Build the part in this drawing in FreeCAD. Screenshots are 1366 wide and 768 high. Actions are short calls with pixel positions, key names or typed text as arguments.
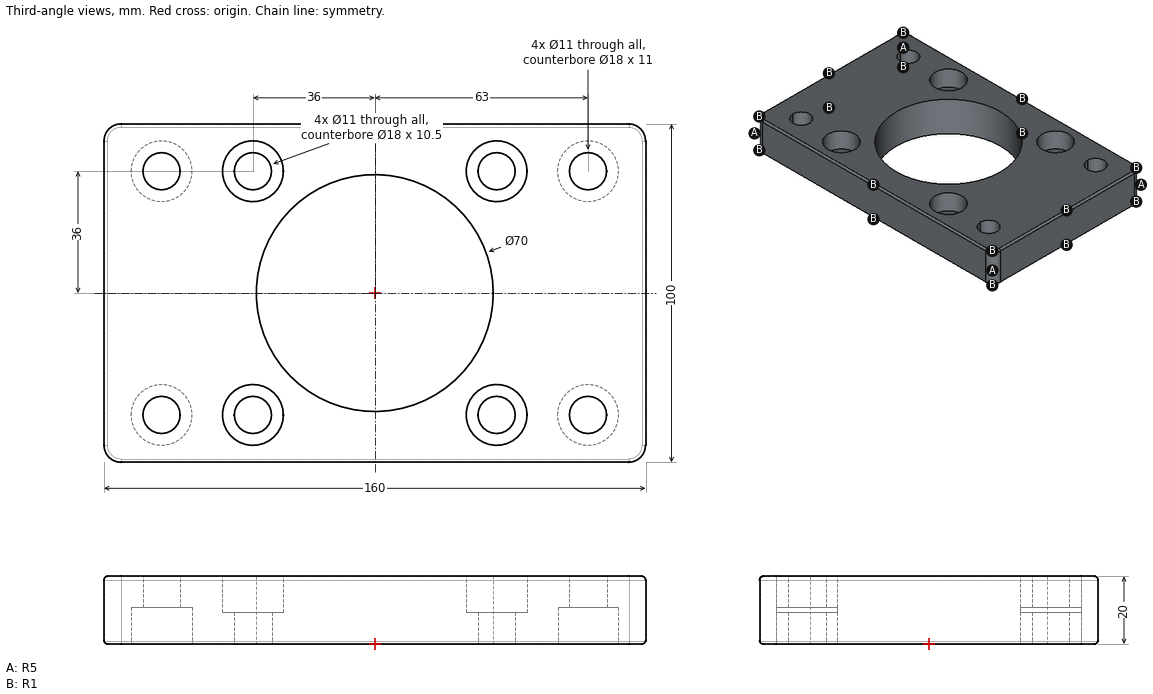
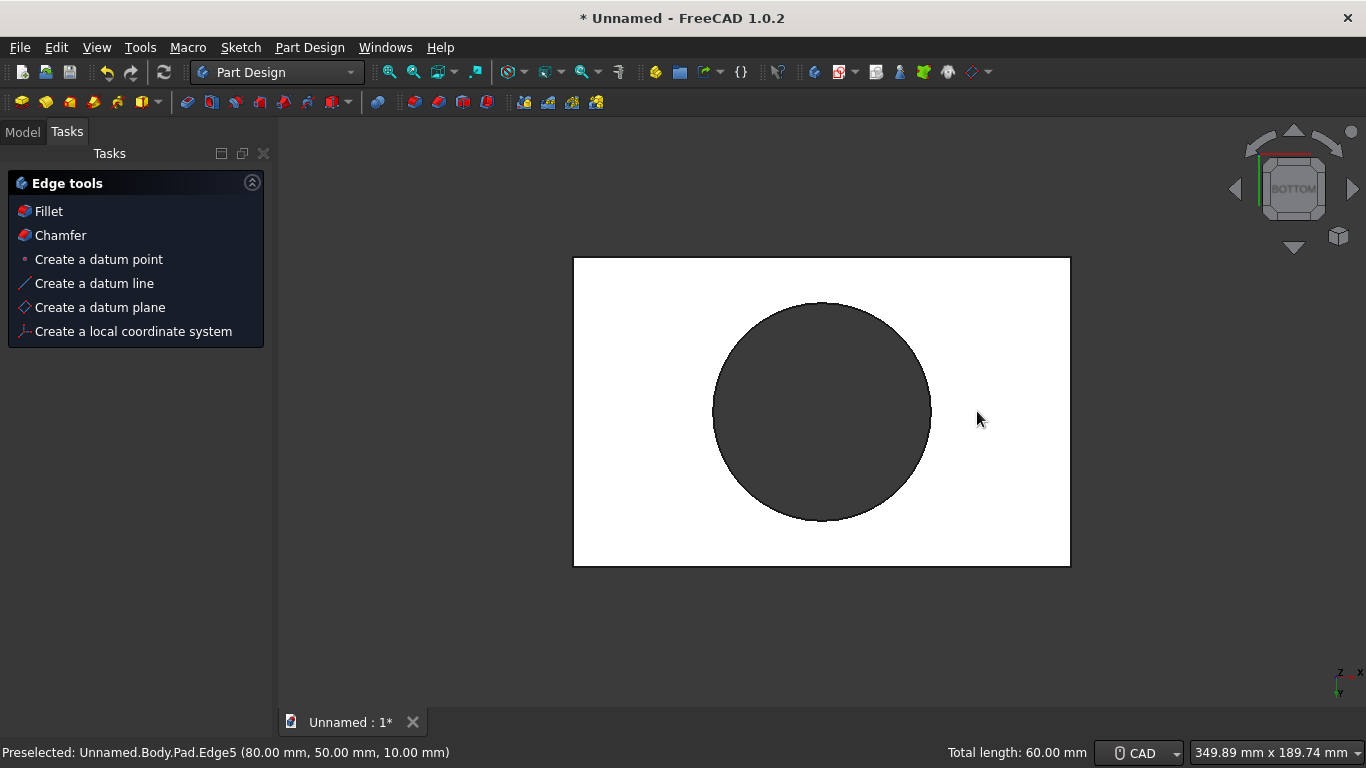
key(4)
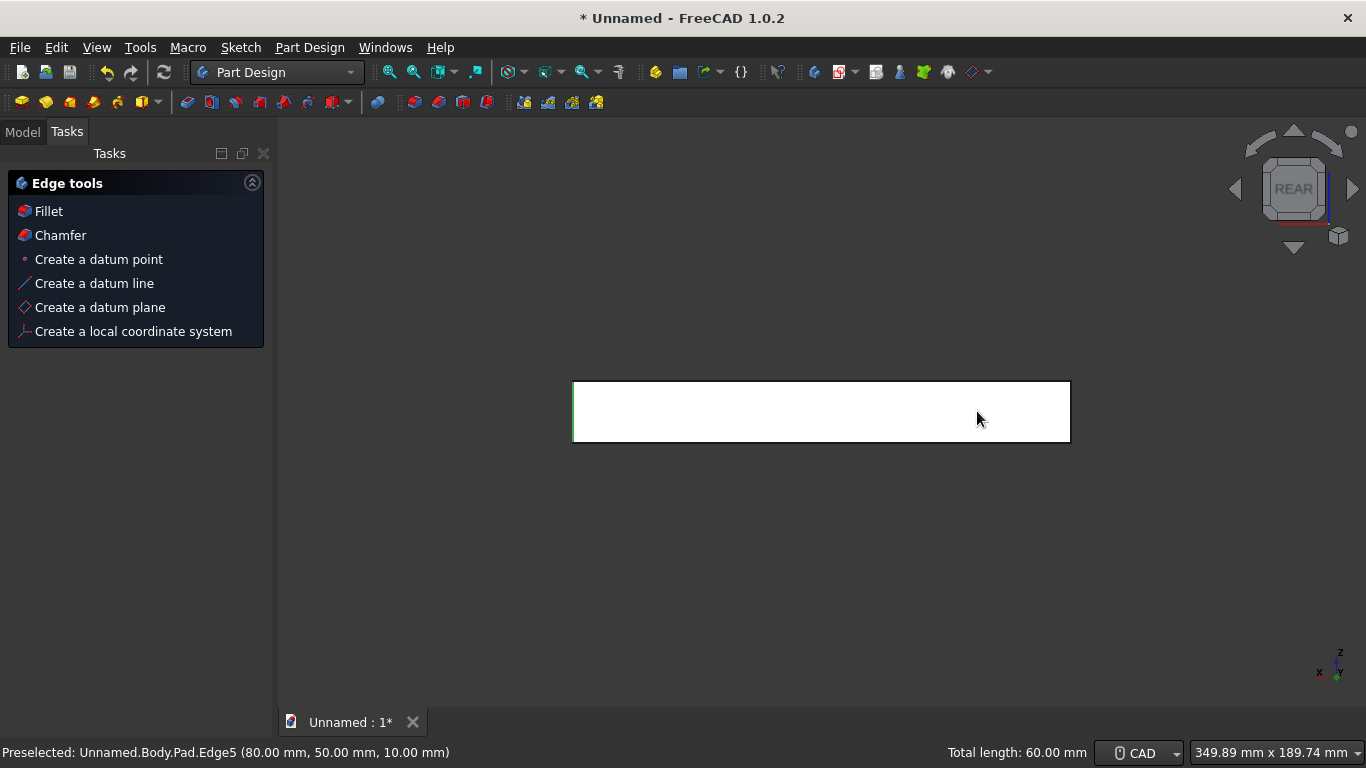
click(1071, 411, ctrl)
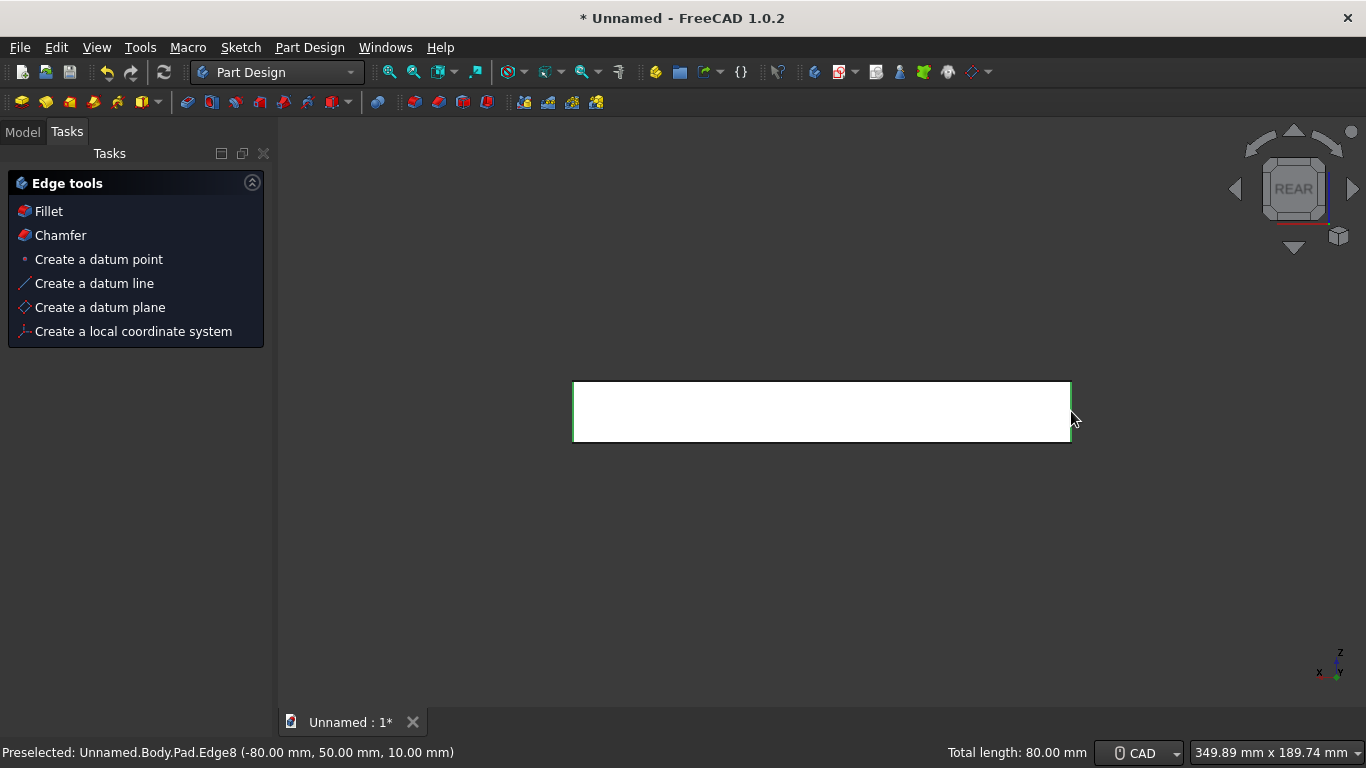
click(416, 102)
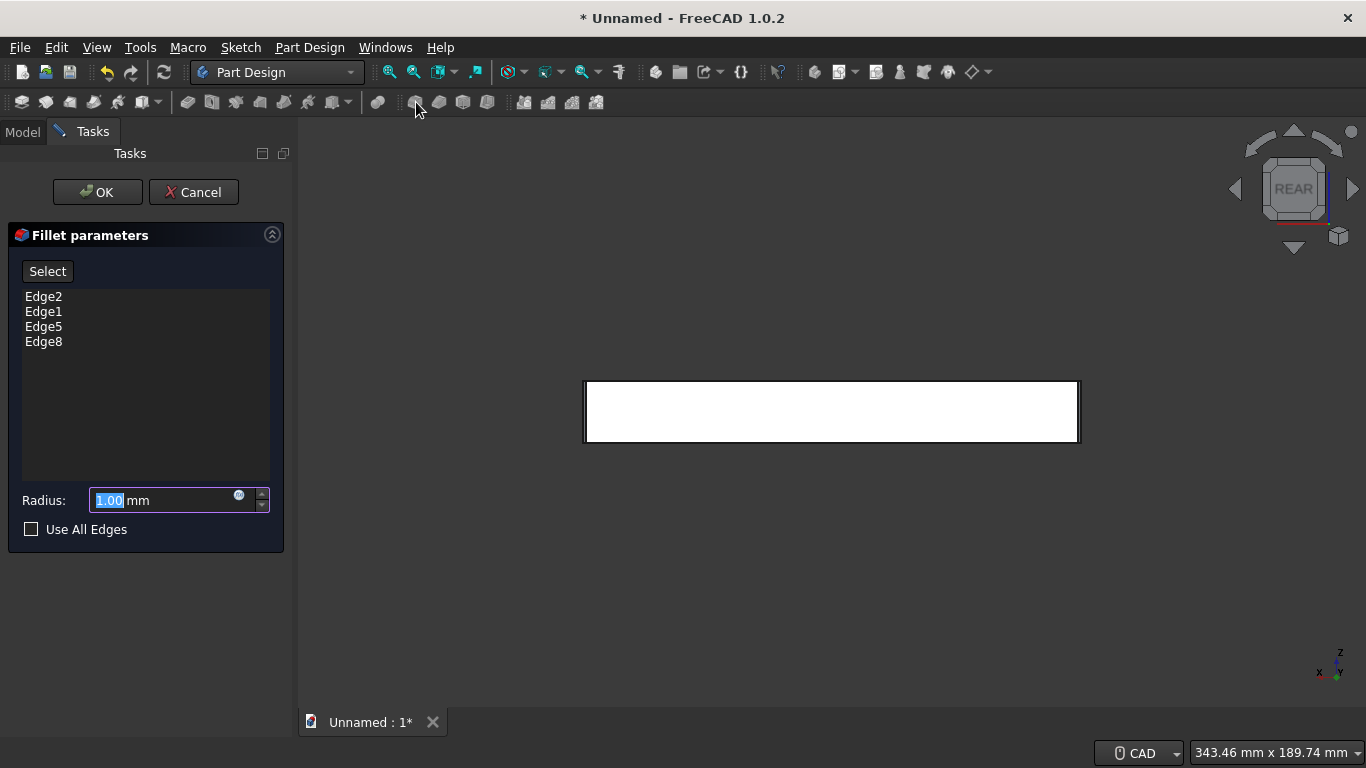
text(5)
key(Tab)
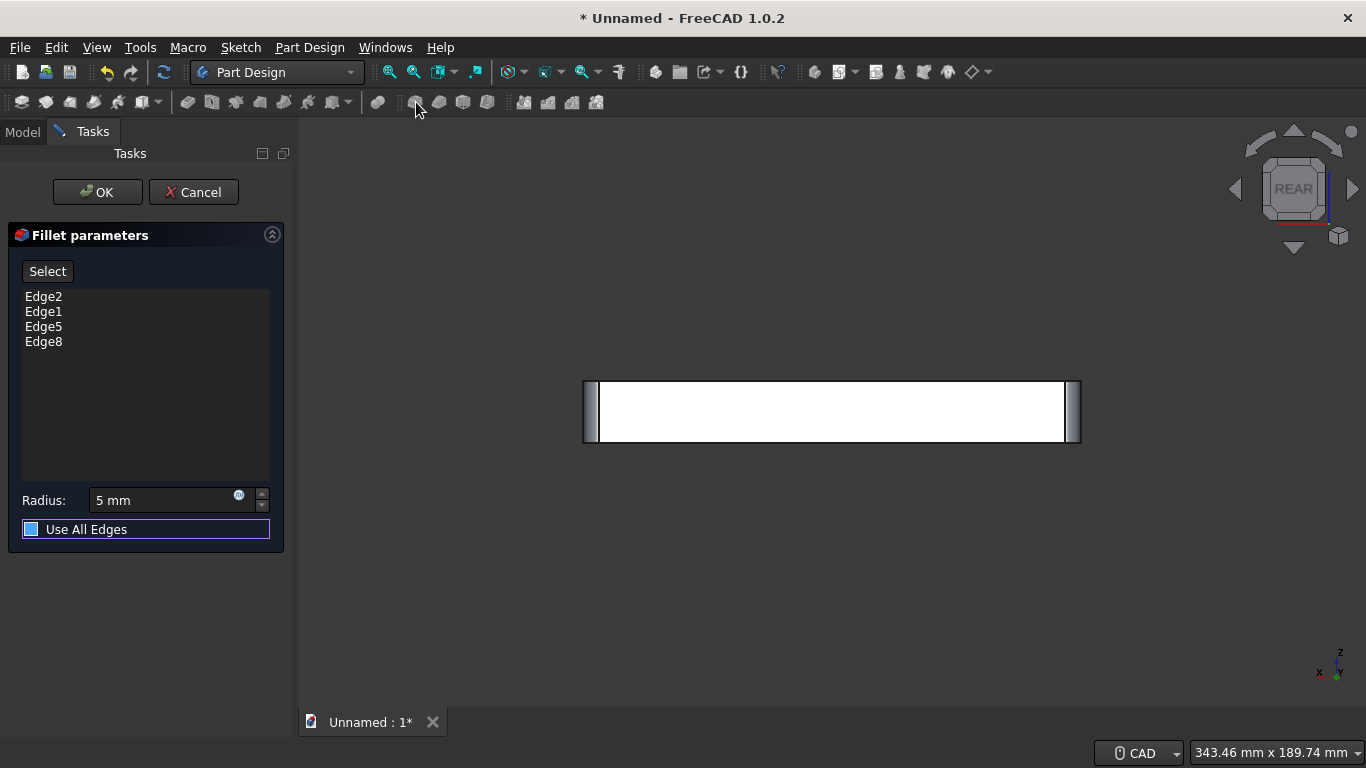
click(98, 192)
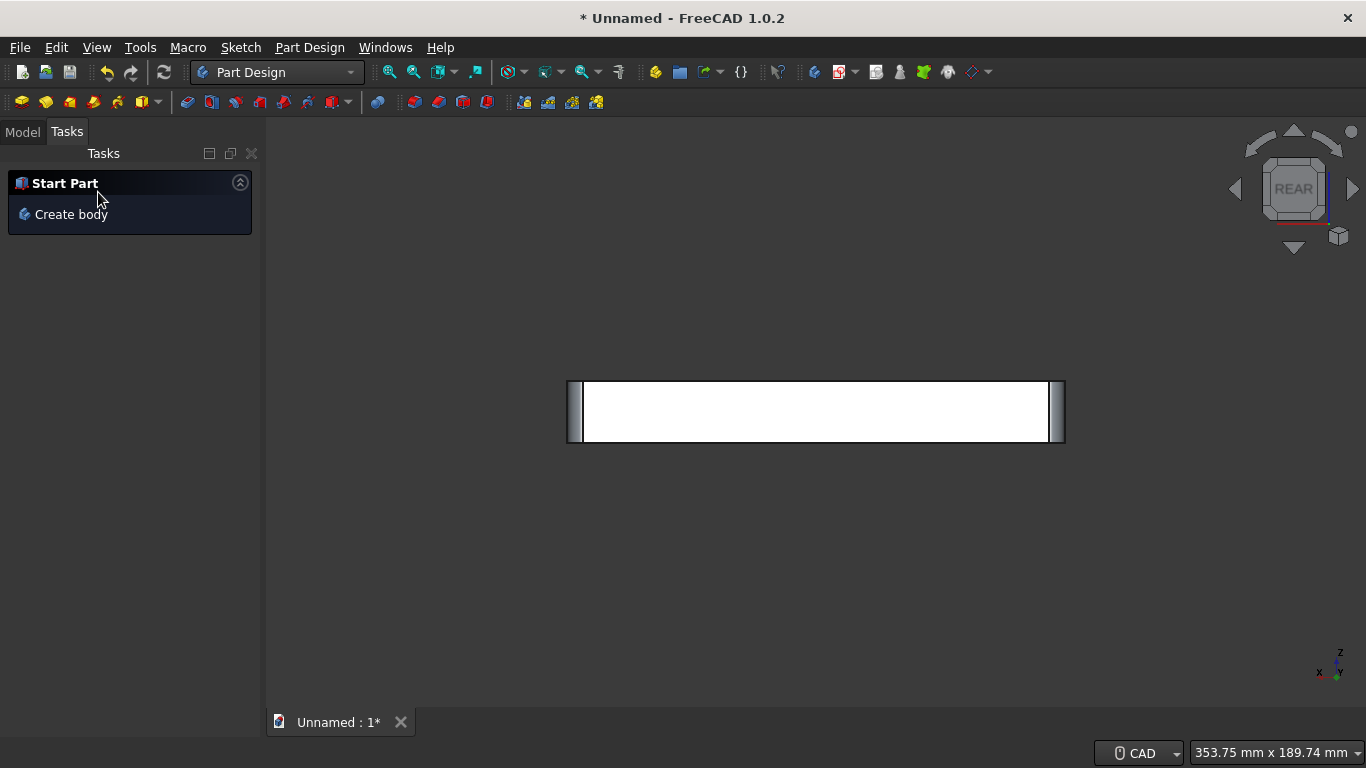
key(0)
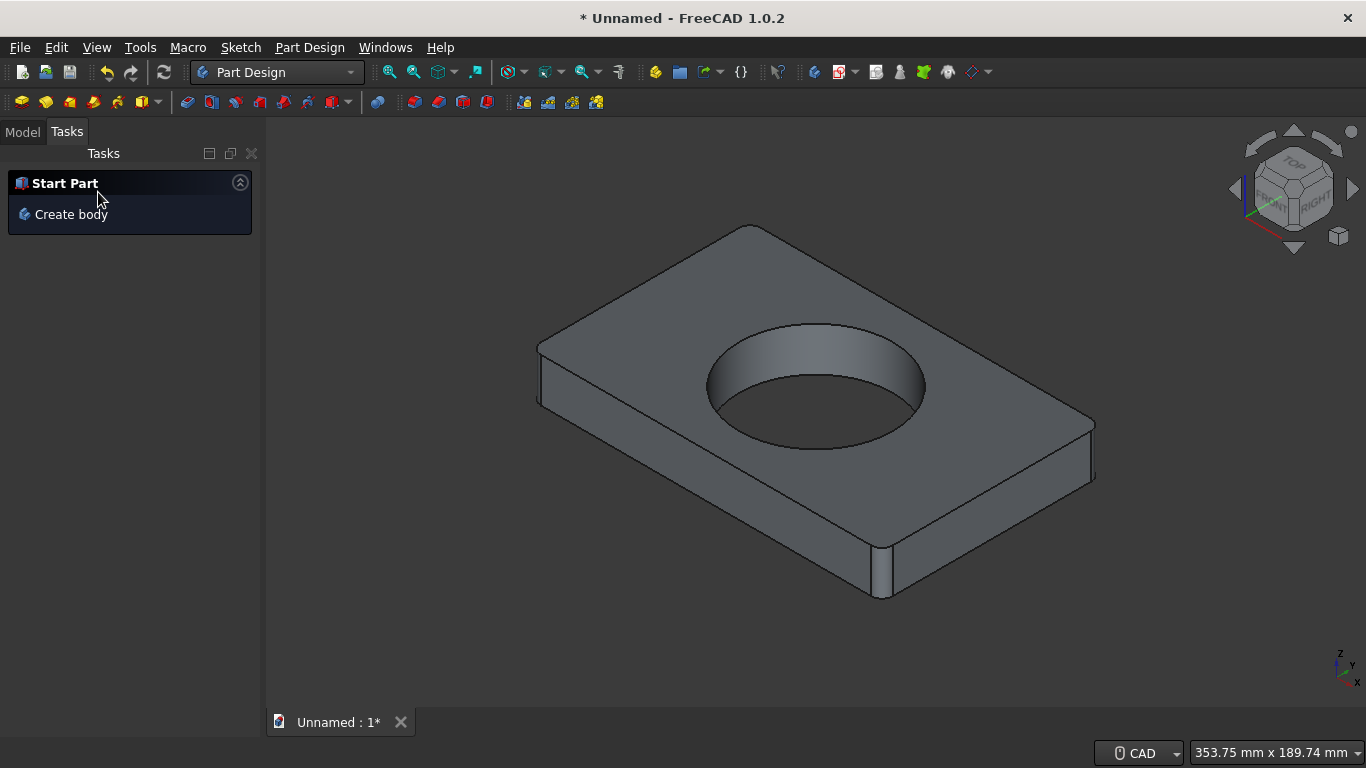
click(653, 364)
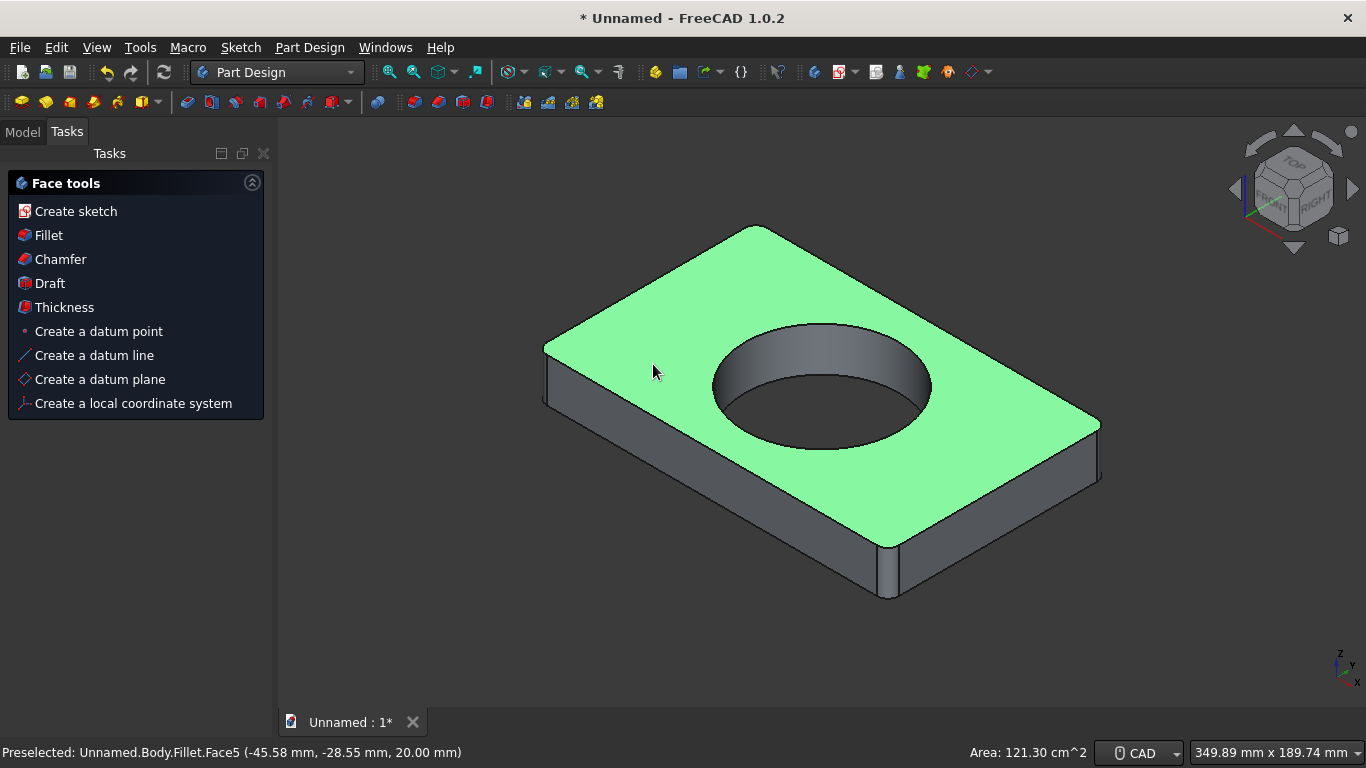
click(840, 72)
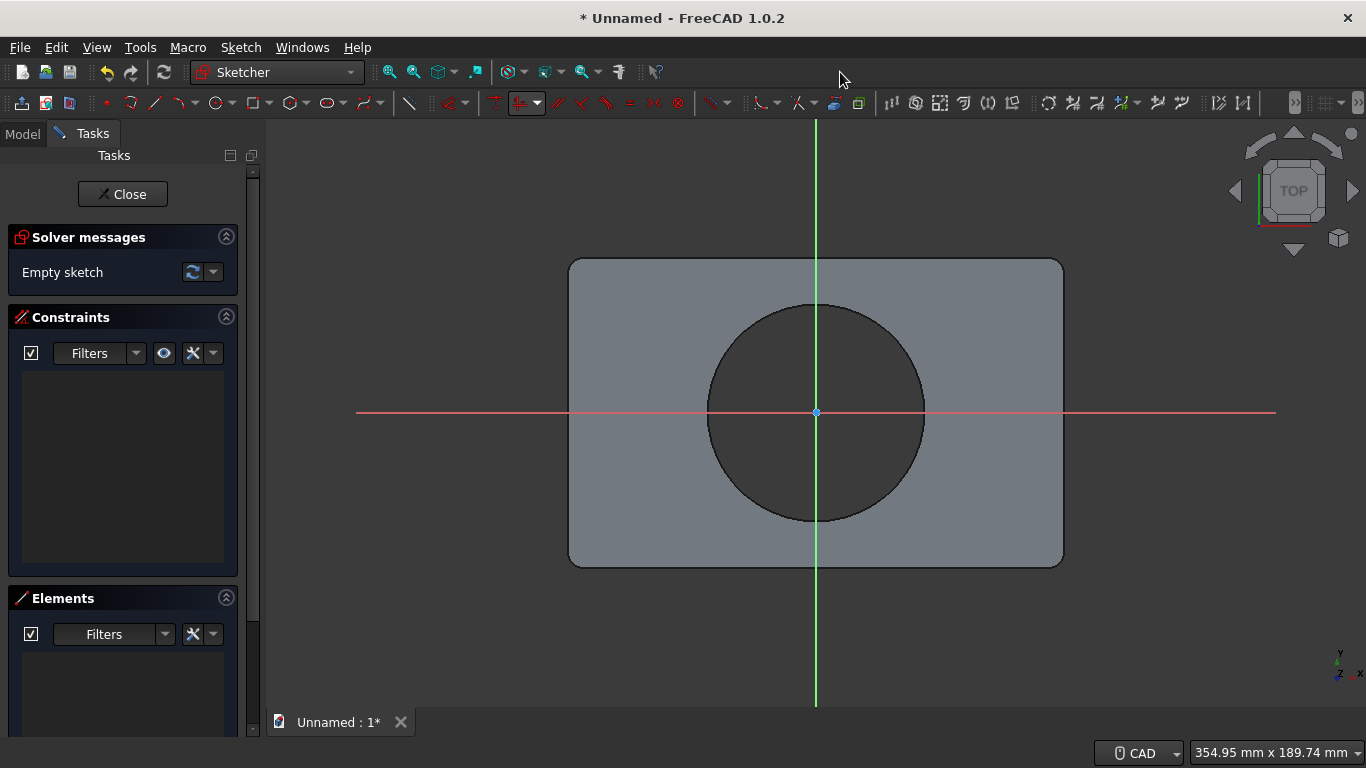
scroll(955, 413, up, 2)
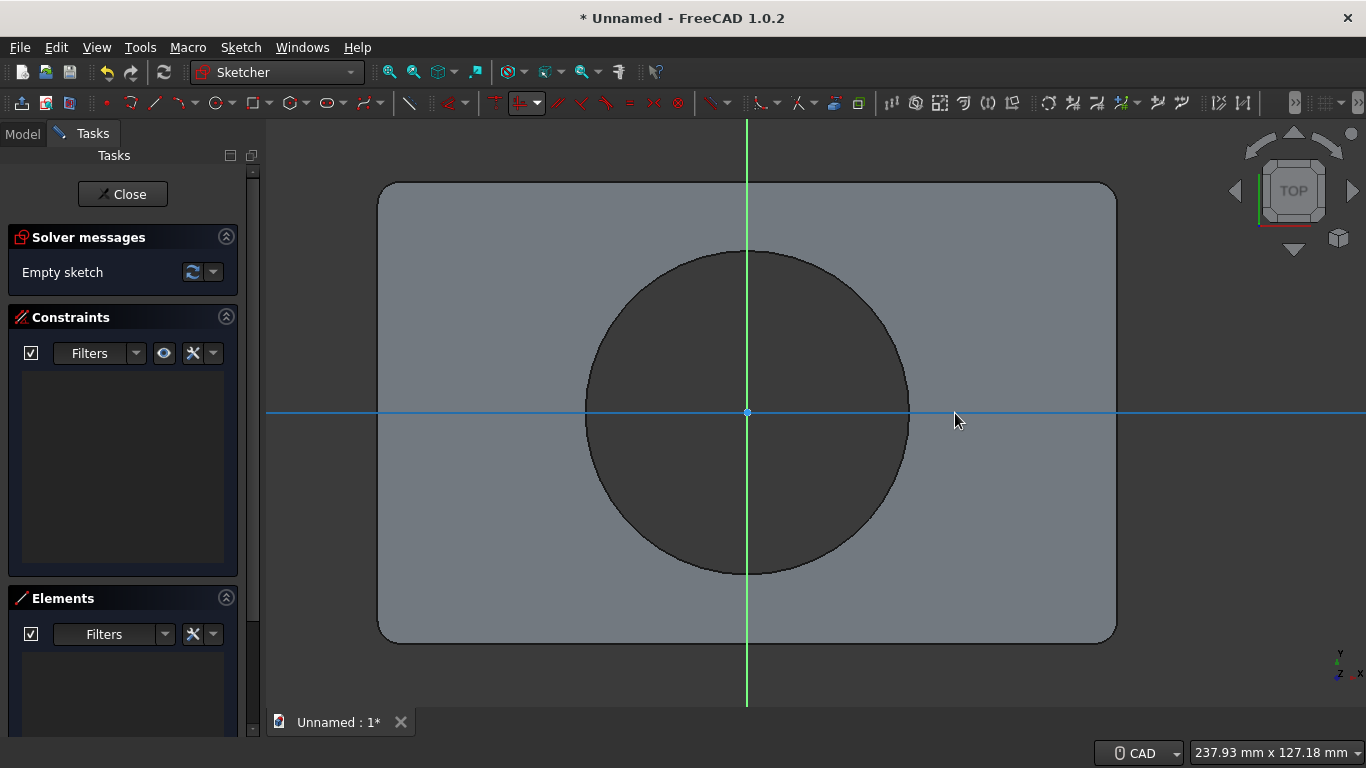
key(g)
key(c)